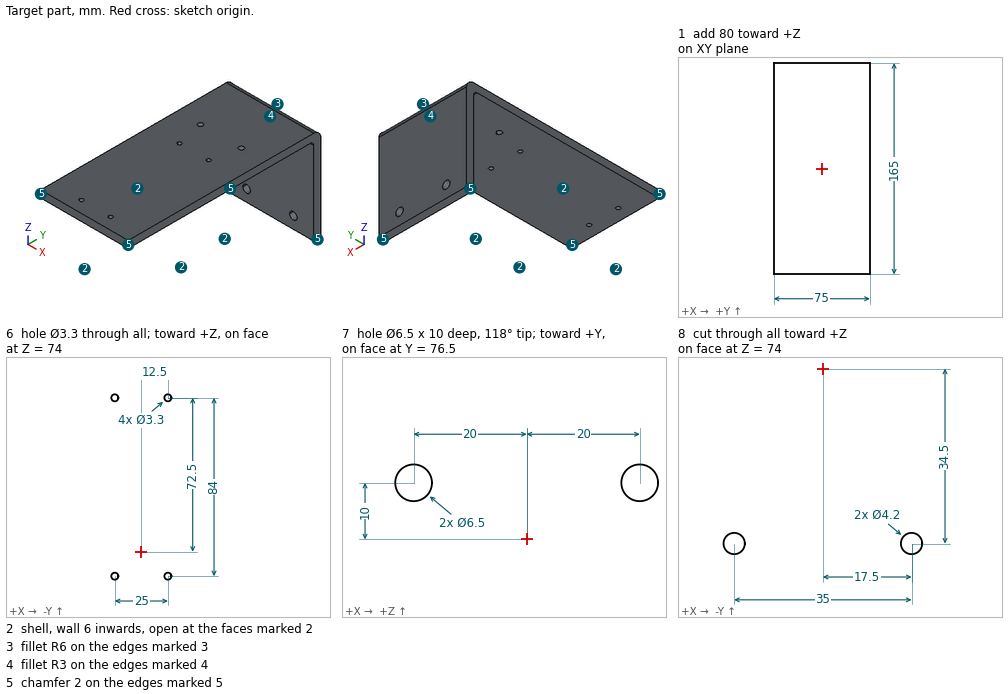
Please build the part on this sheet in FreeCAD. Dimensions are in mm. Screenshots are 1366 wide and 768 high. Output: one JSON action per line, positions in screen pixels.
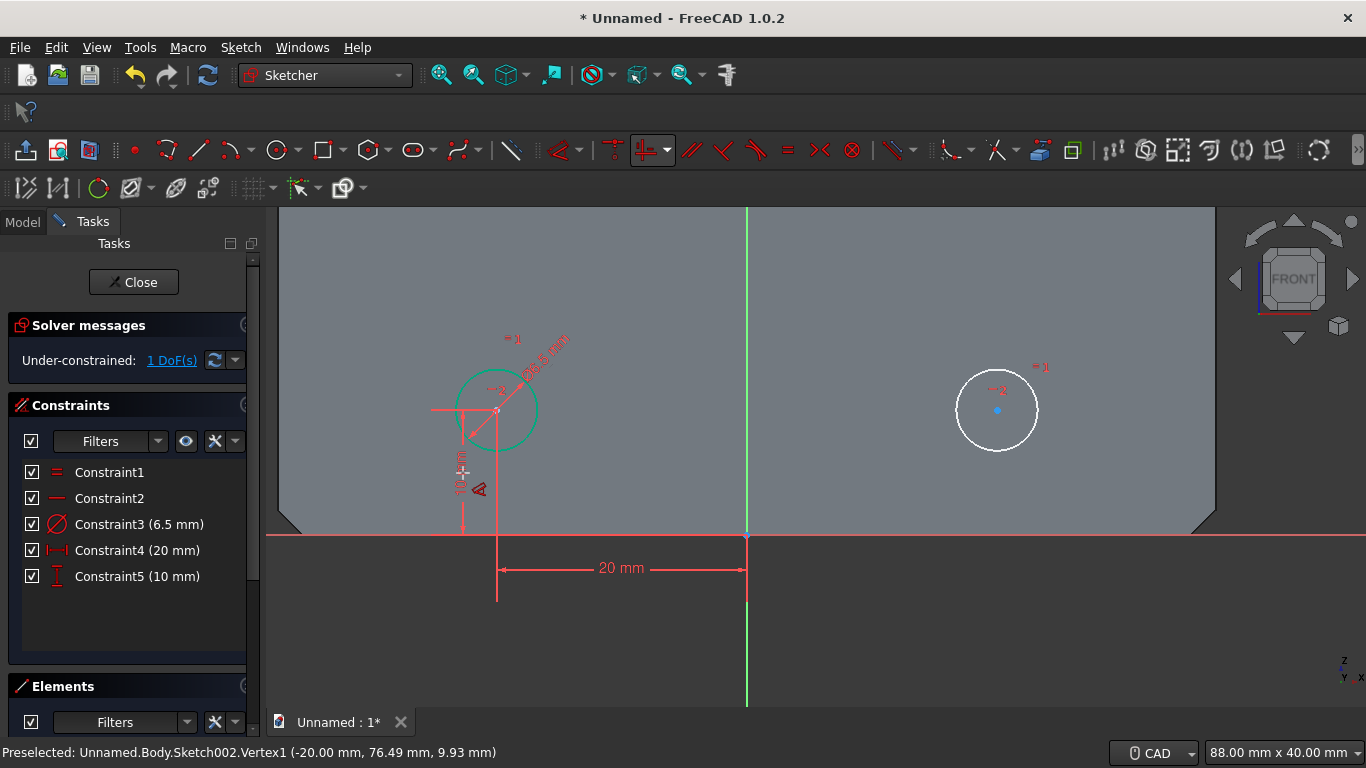
{"action": "left_click", "coordinate": [997, 410]}
{"action": "left_click", "coordinate": [872, 569]}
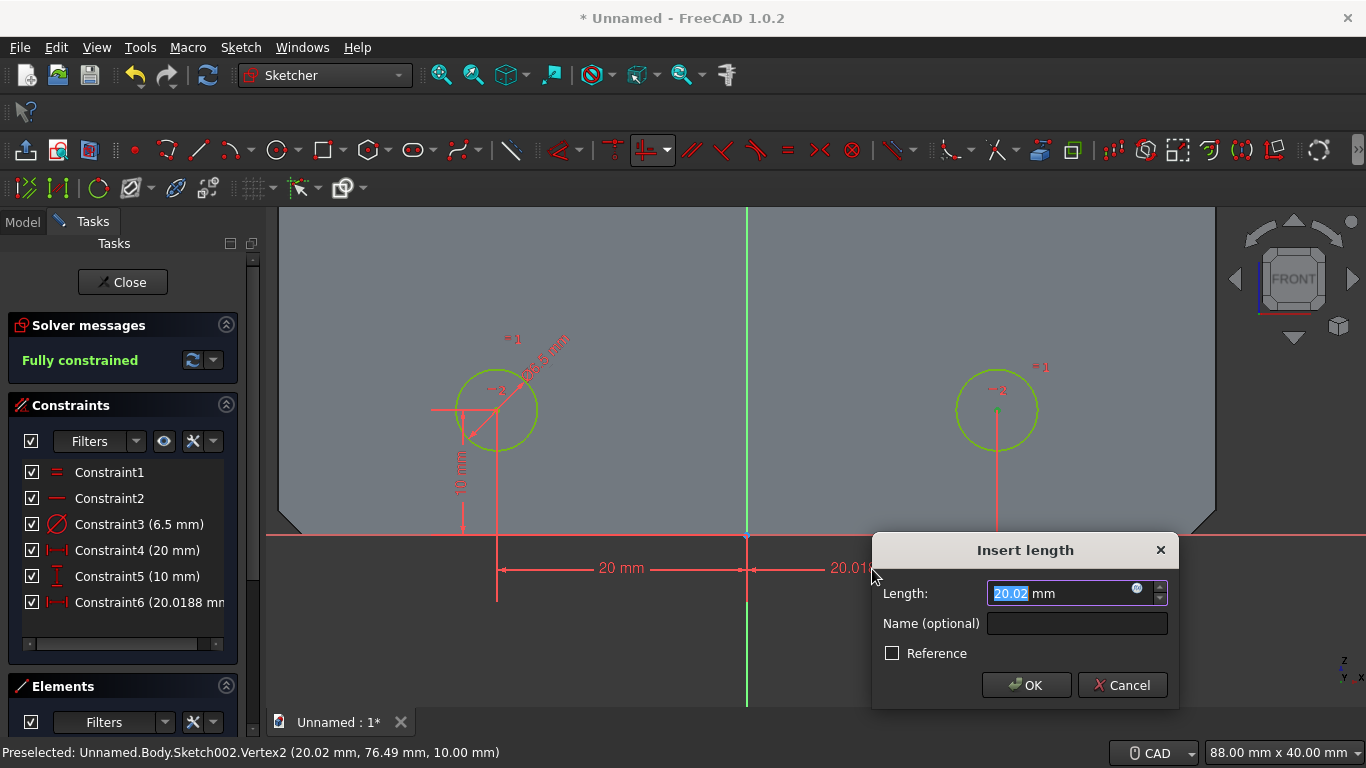
{"action": "type", "text": "20"}
{"action": "key", "text": "Return"}
{"action": "key", "text": "Escape"}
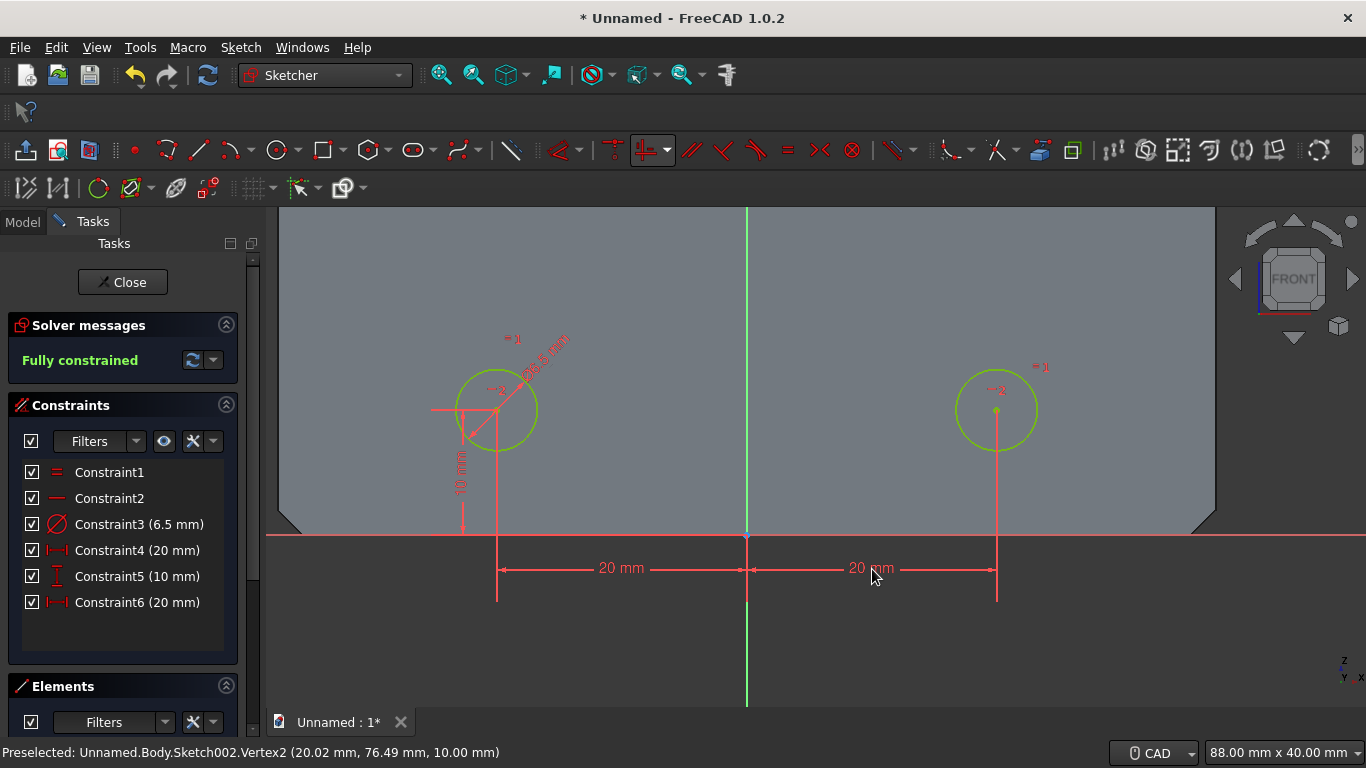
{"action": "left_click", "coordinate": [123, 282]}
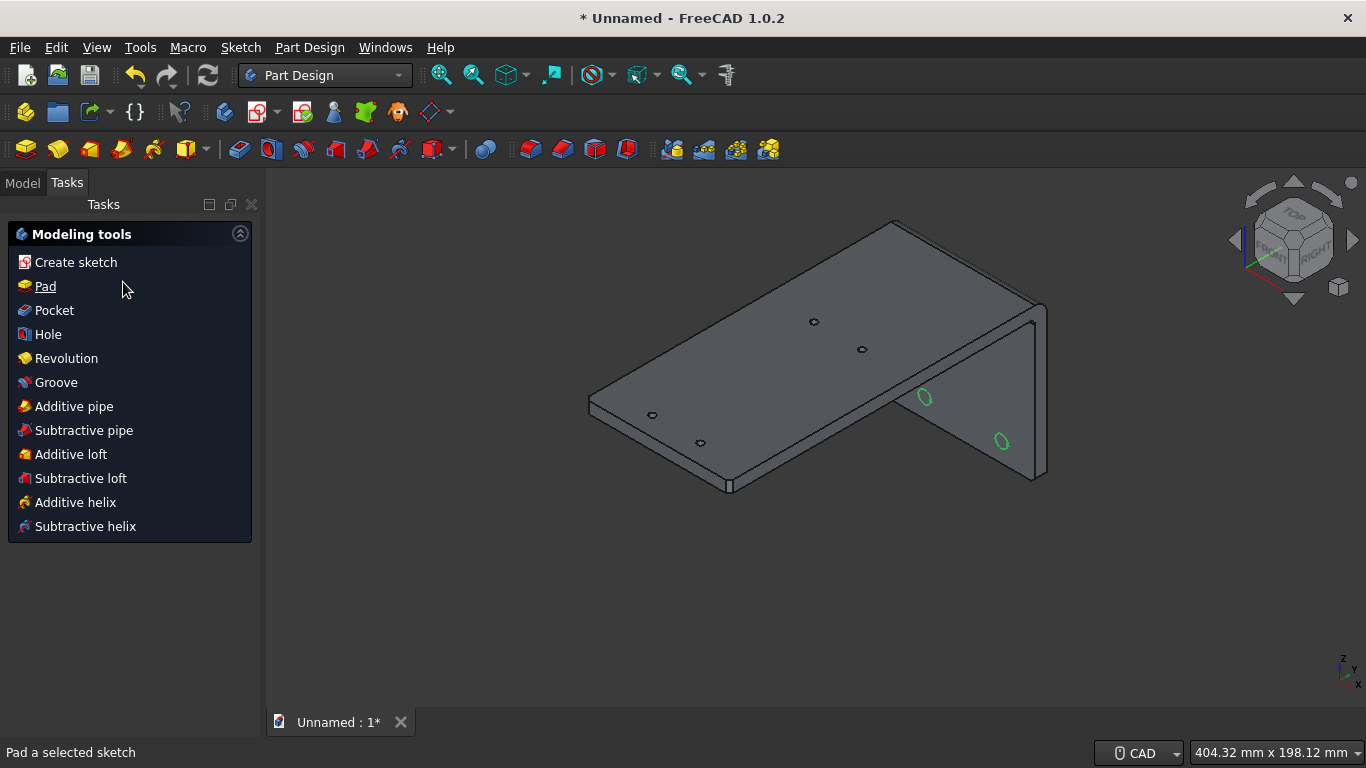
{"action": "left_click", "coordinate": [272, 150]}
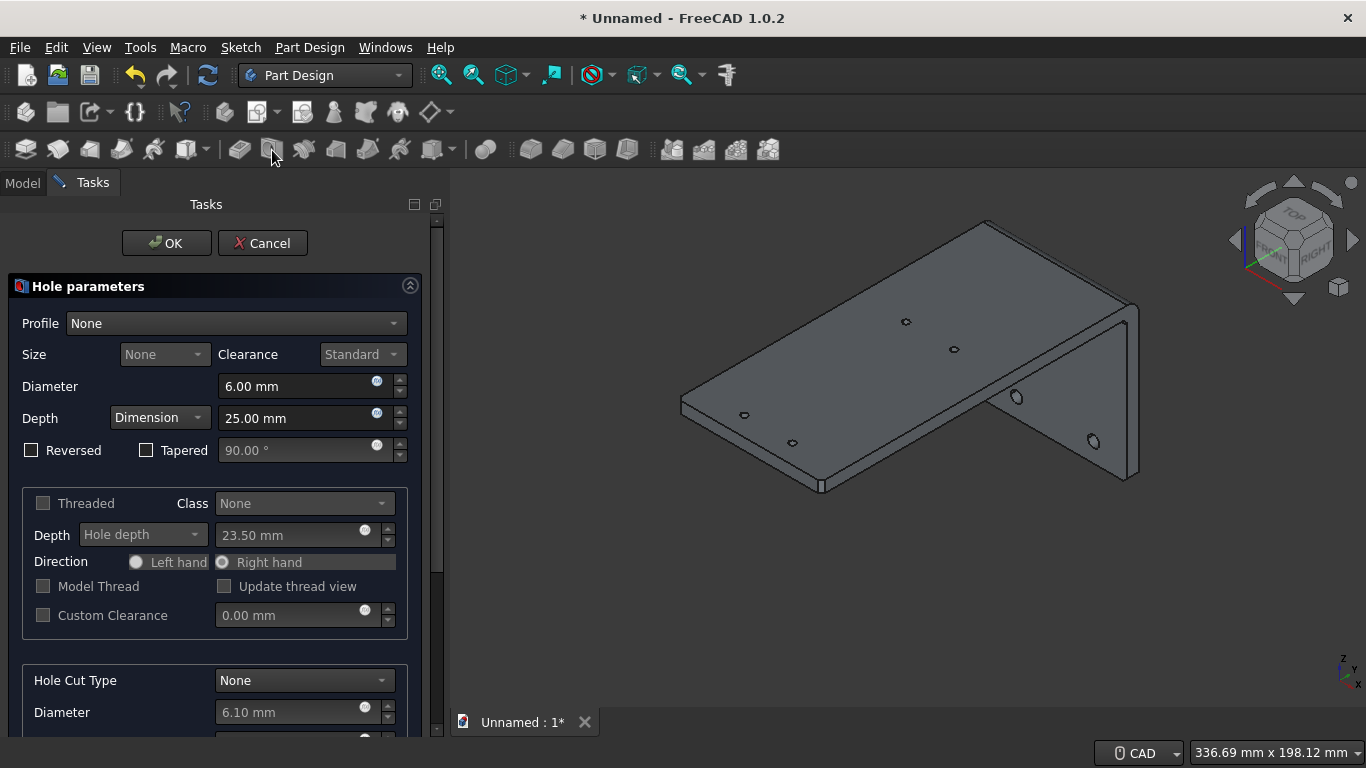
{"action": "triple_click", "coordinate": [305, 386]}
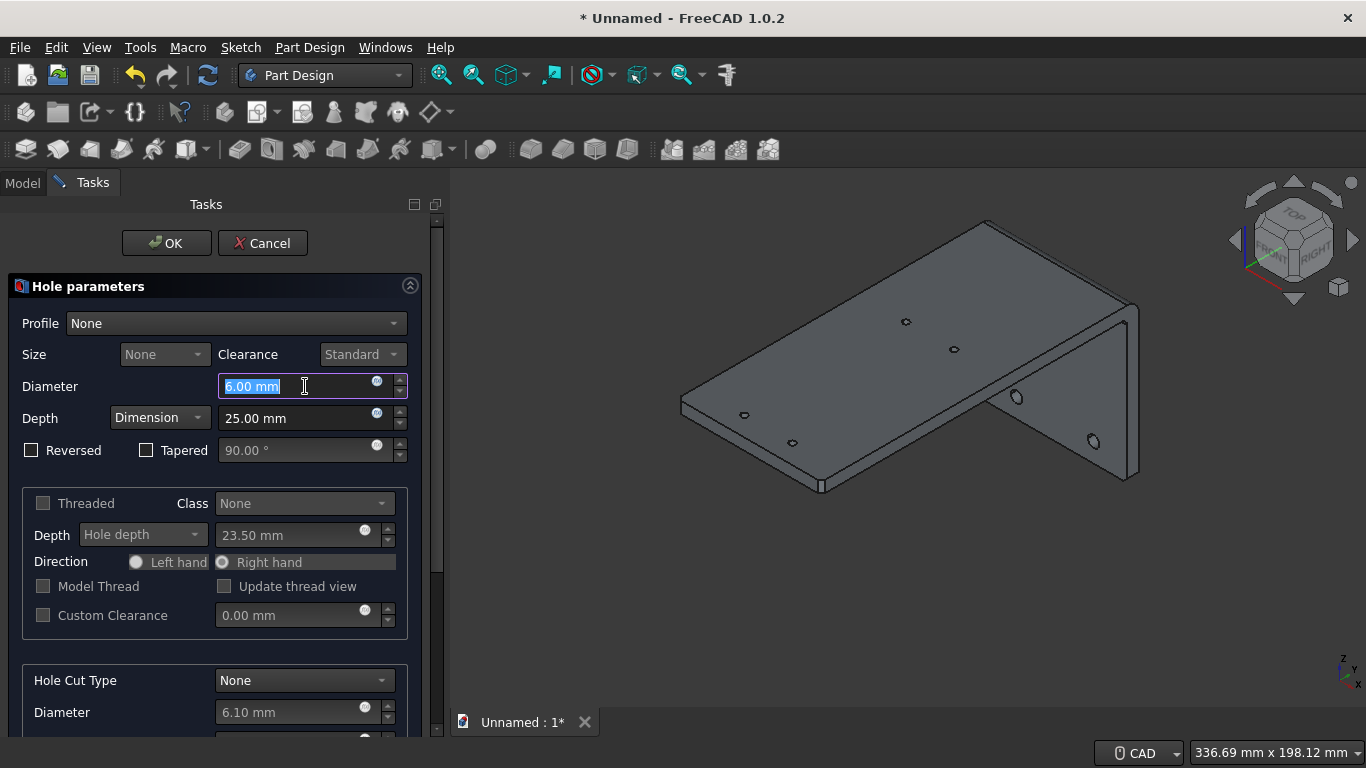
{"action": "type", "text": "6.5"}
{"action": "key", "text": "Tab"}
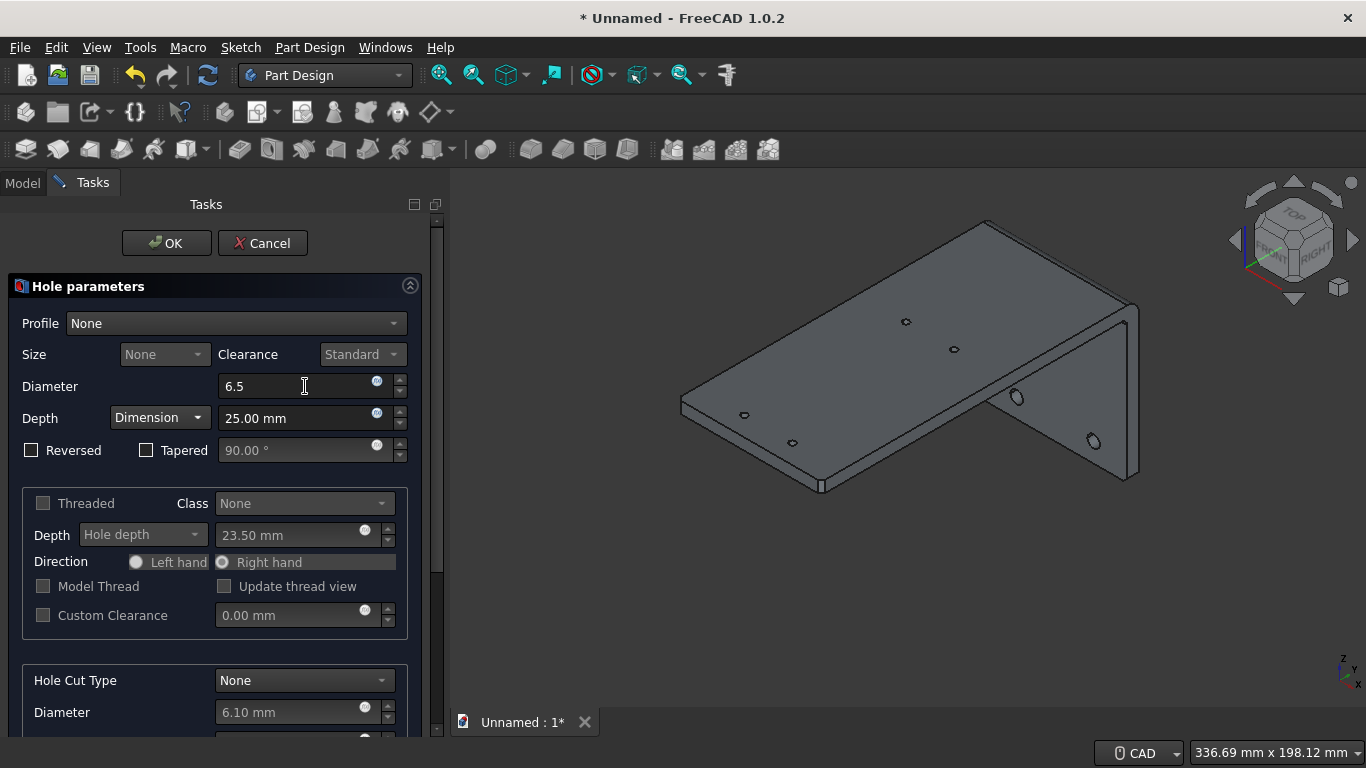
{"action": "triple_click", "coordinate": [305, 418]}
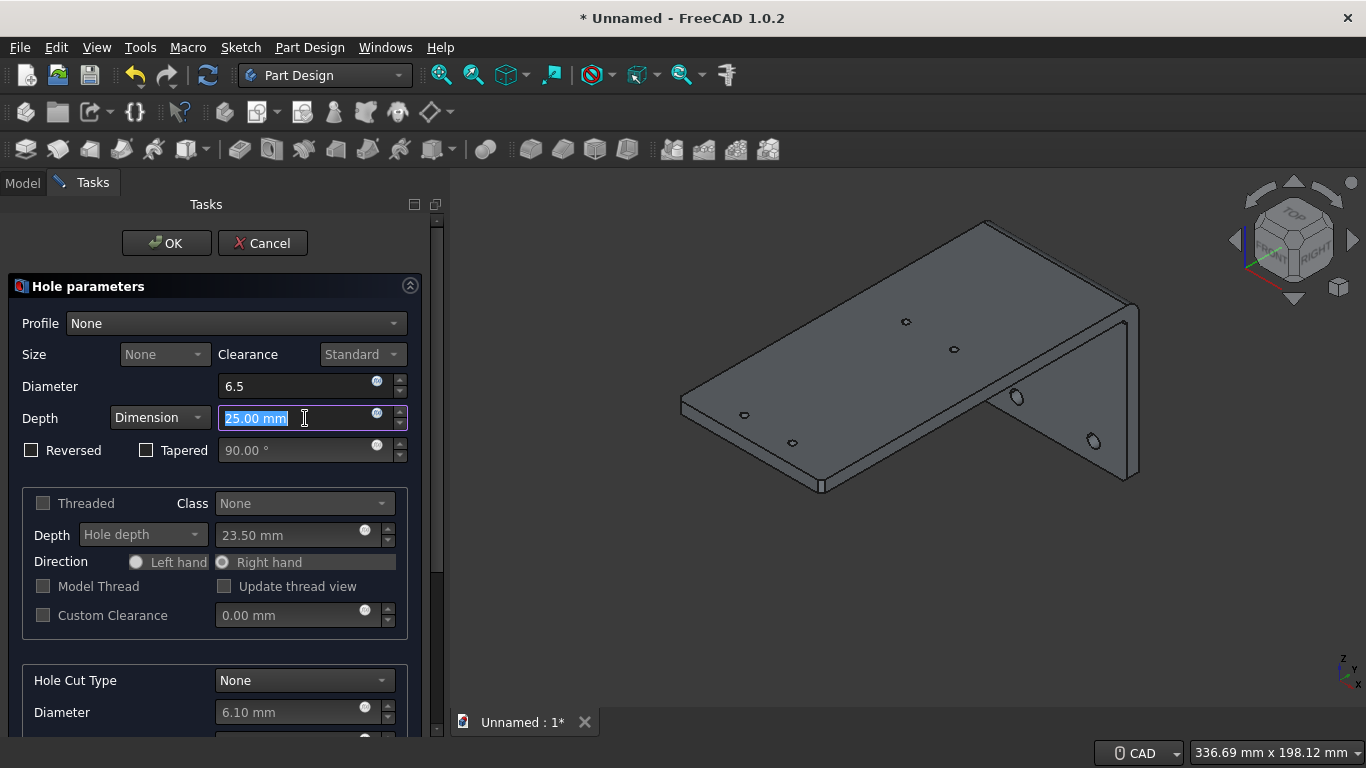
{"action": "type", "text": "10"}
{"action": "key", "text": "Tab"}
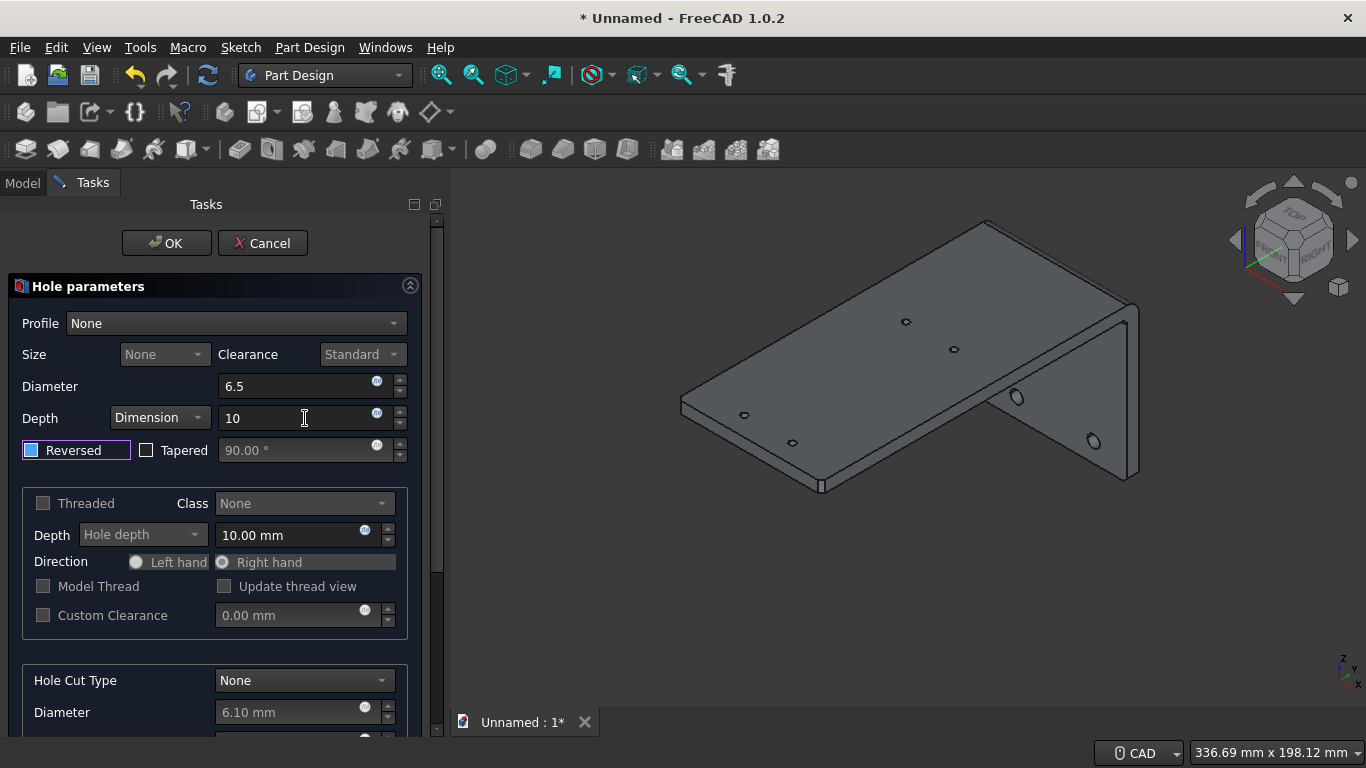
{"action": "left_click", "coordinate": [167, 243]}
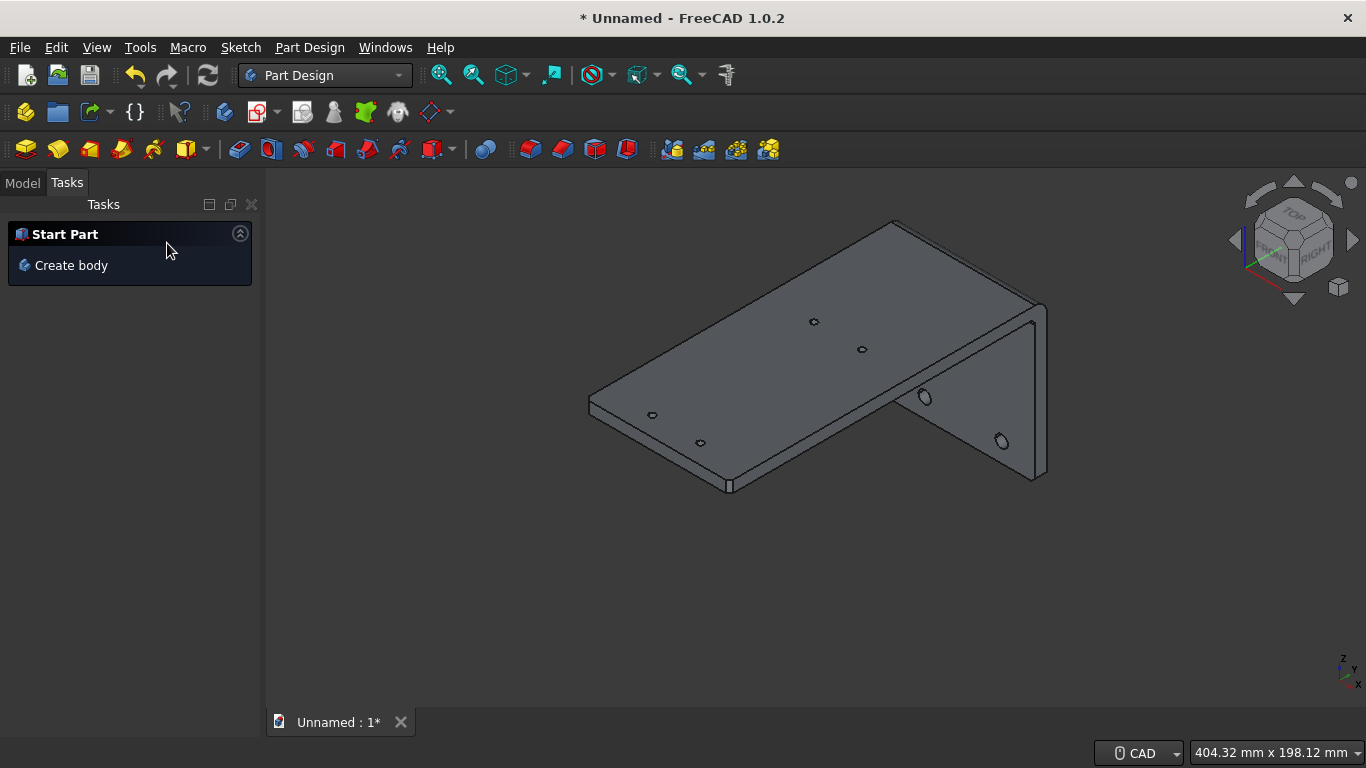
{"action": "key", "text": "5"}